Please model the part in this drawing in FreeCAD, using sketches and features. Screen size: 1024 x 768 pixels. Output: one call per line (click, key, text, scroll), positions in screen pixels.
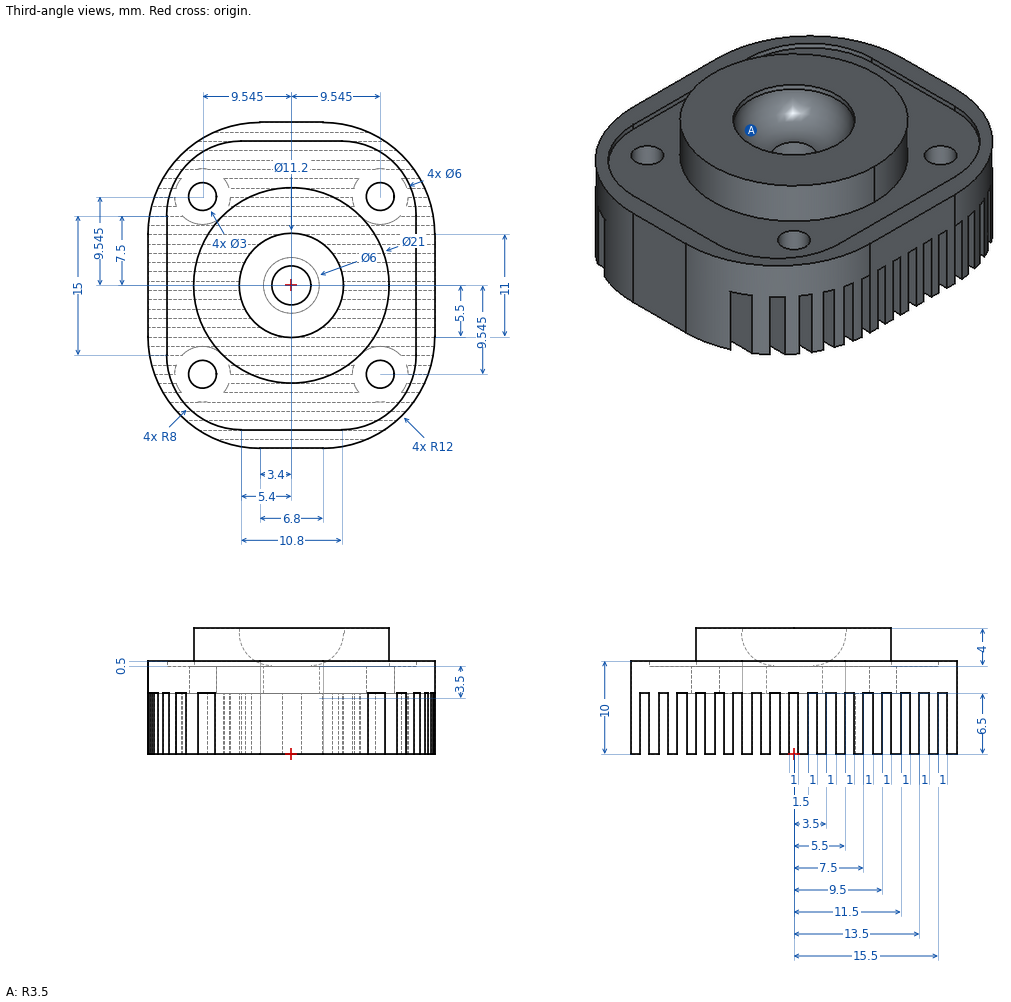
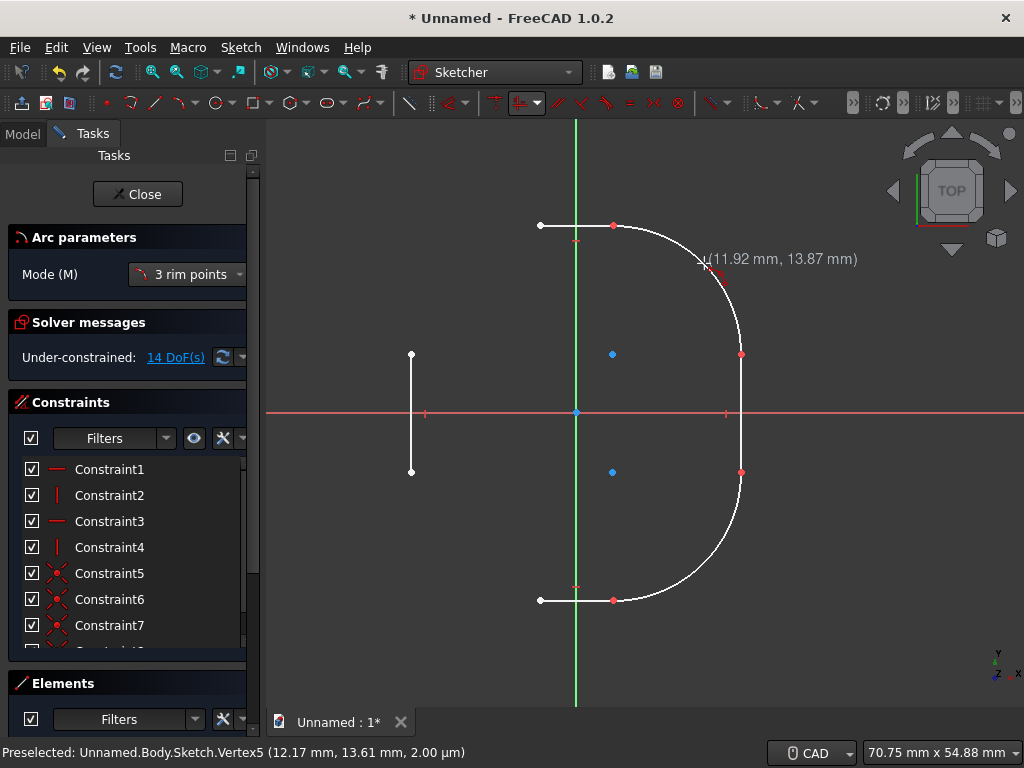
click(540, 226)
click(411, 355)
click(449, 263)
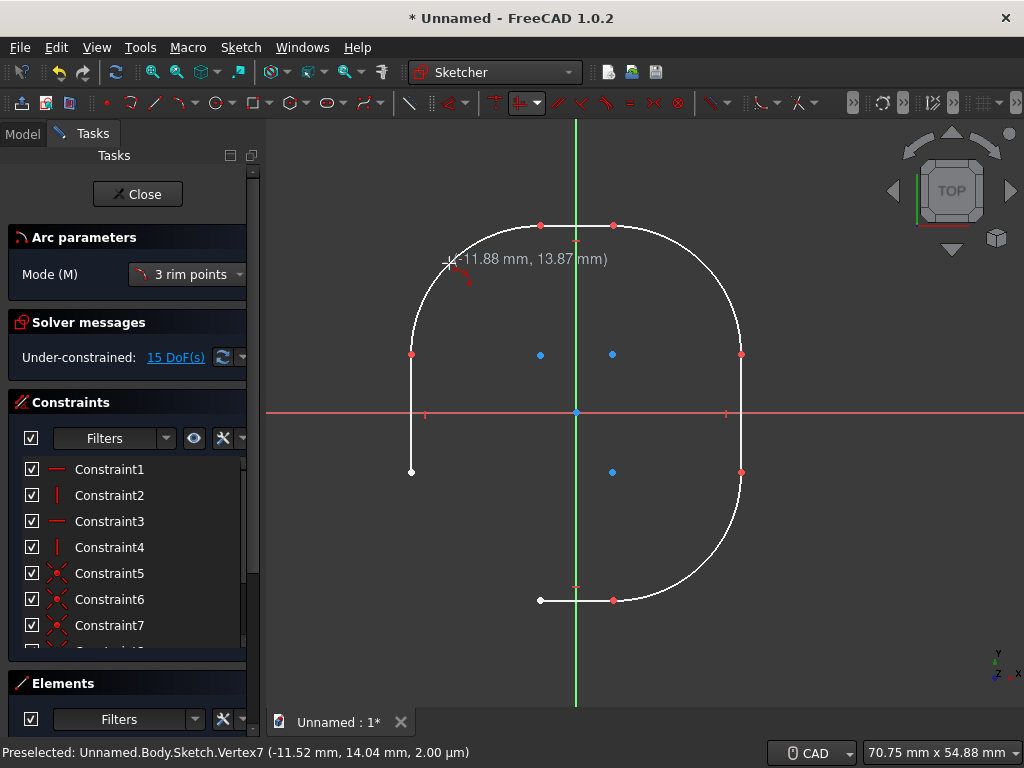
click(411, 473)
click(540, 601)
click(449, 562)
key(Escape)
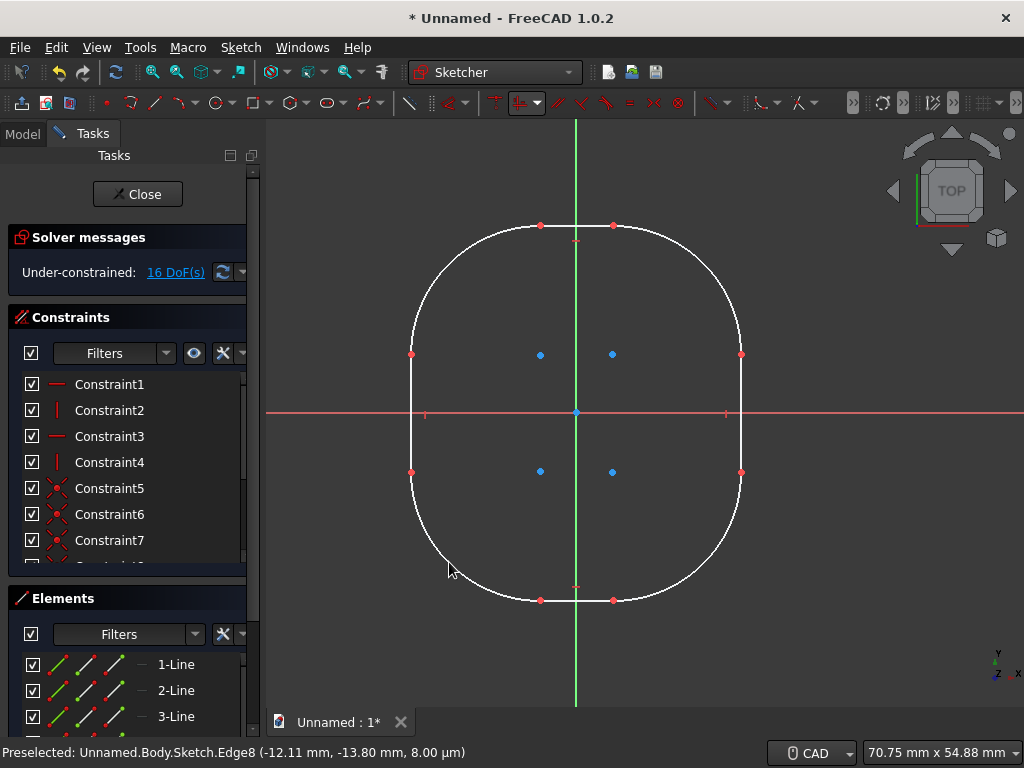
click(562, 601)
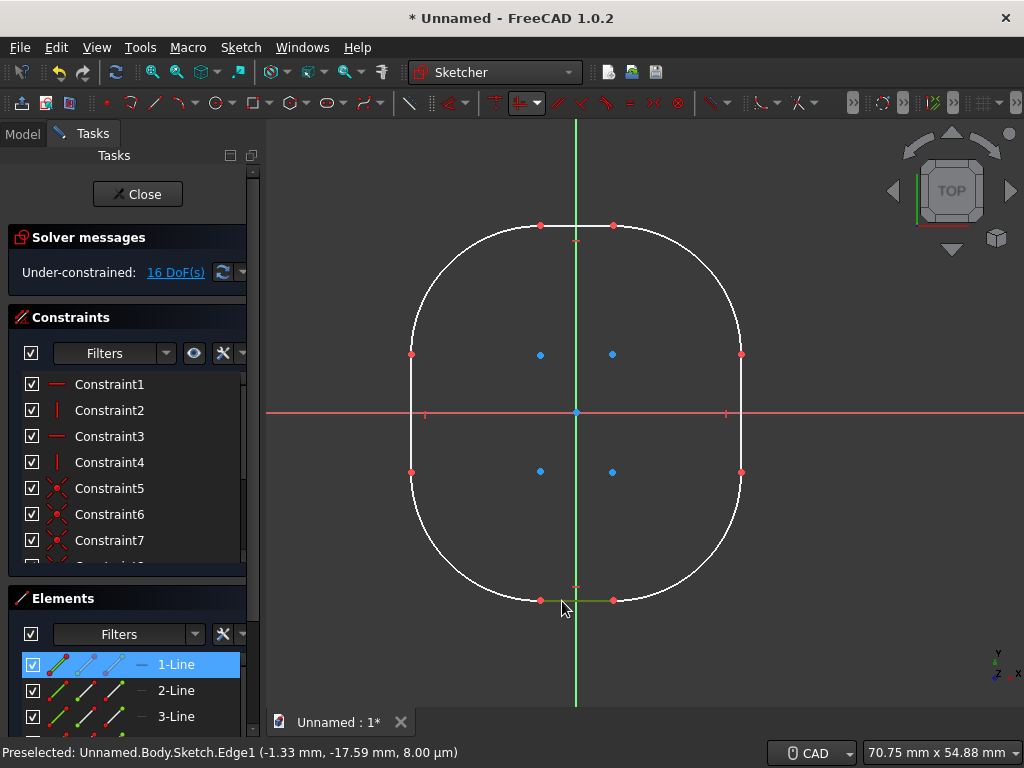
click(671, 587)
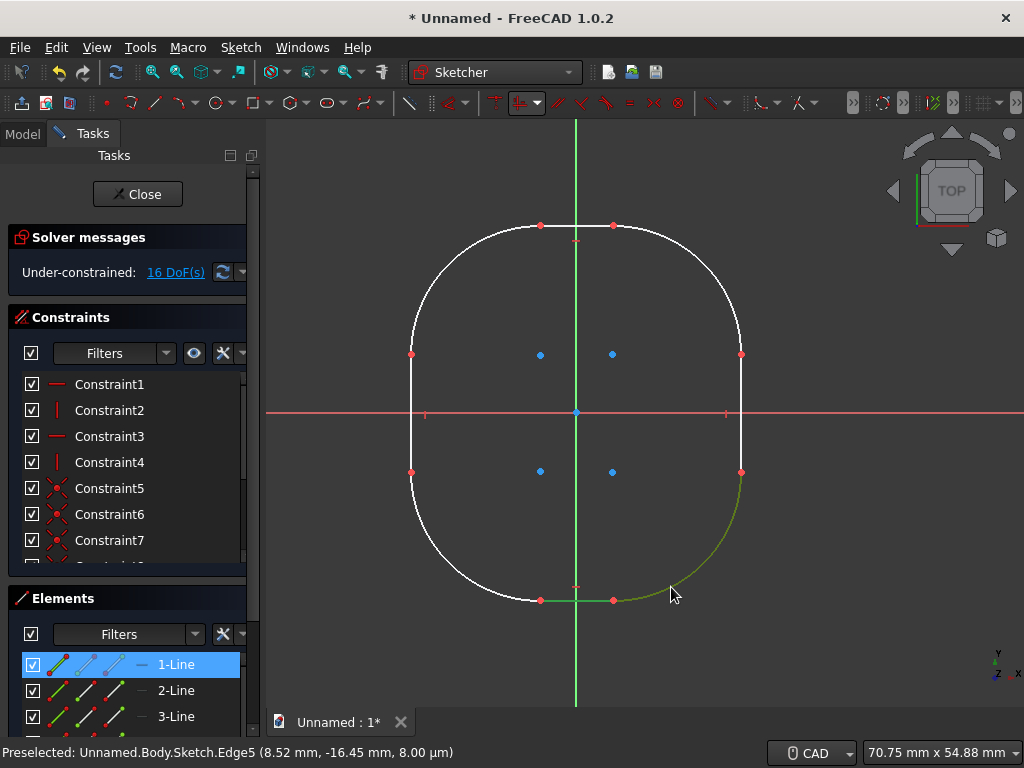
key(t)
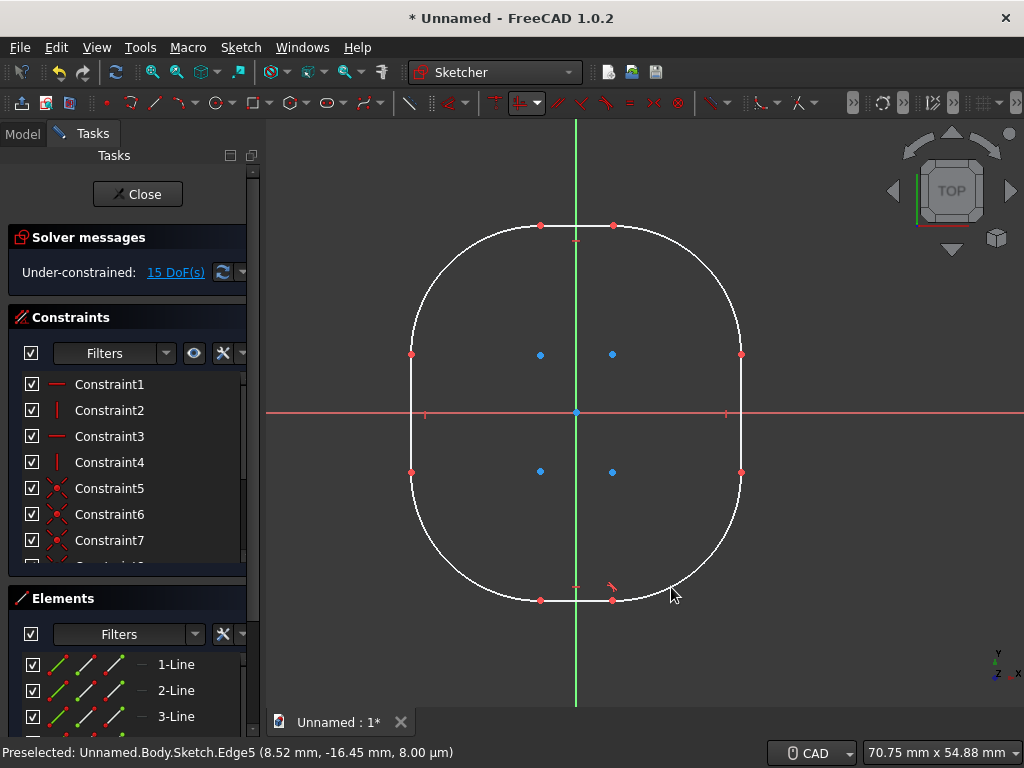
click(562, 601)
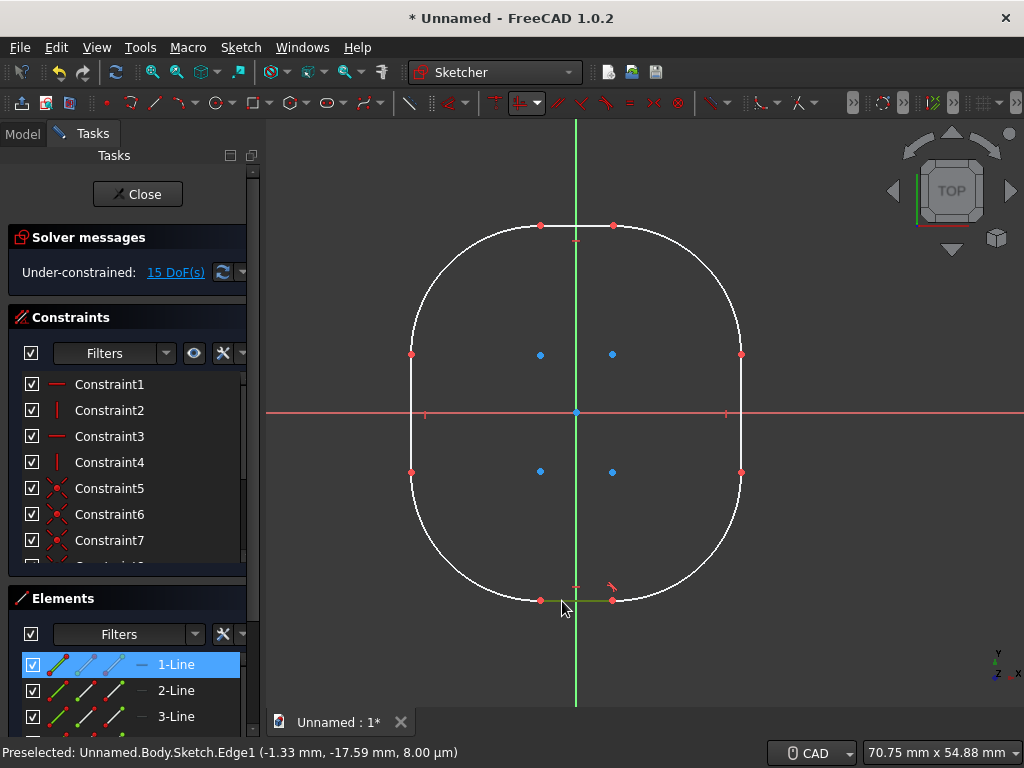
click(426, 531)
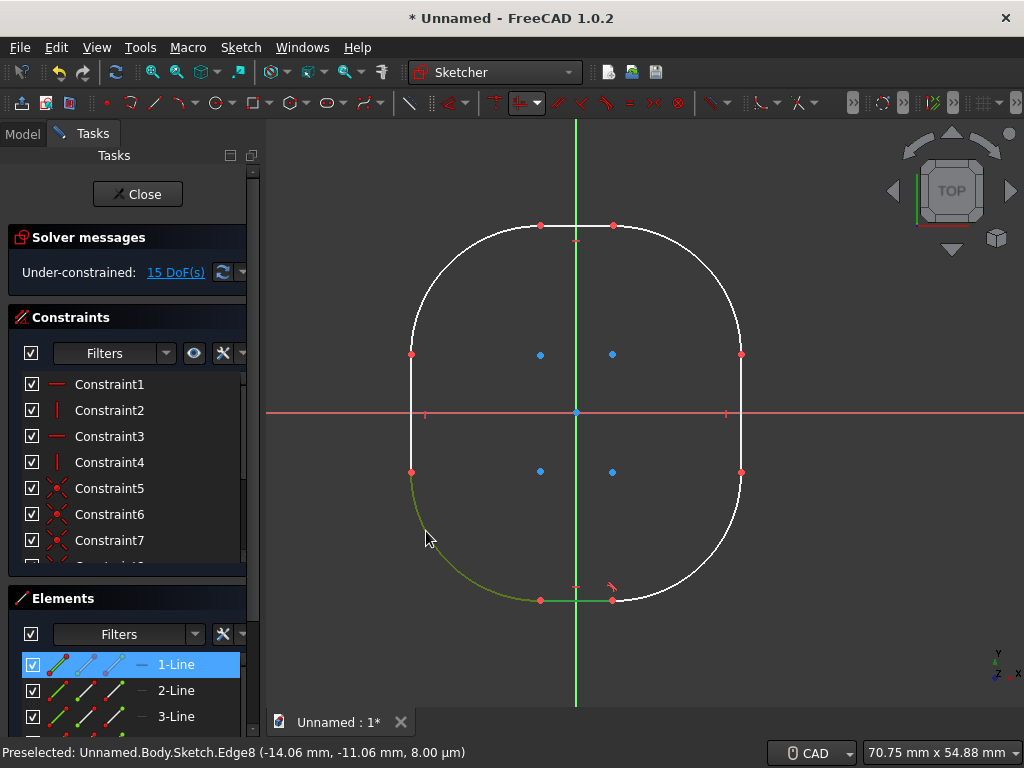
click(606, 104)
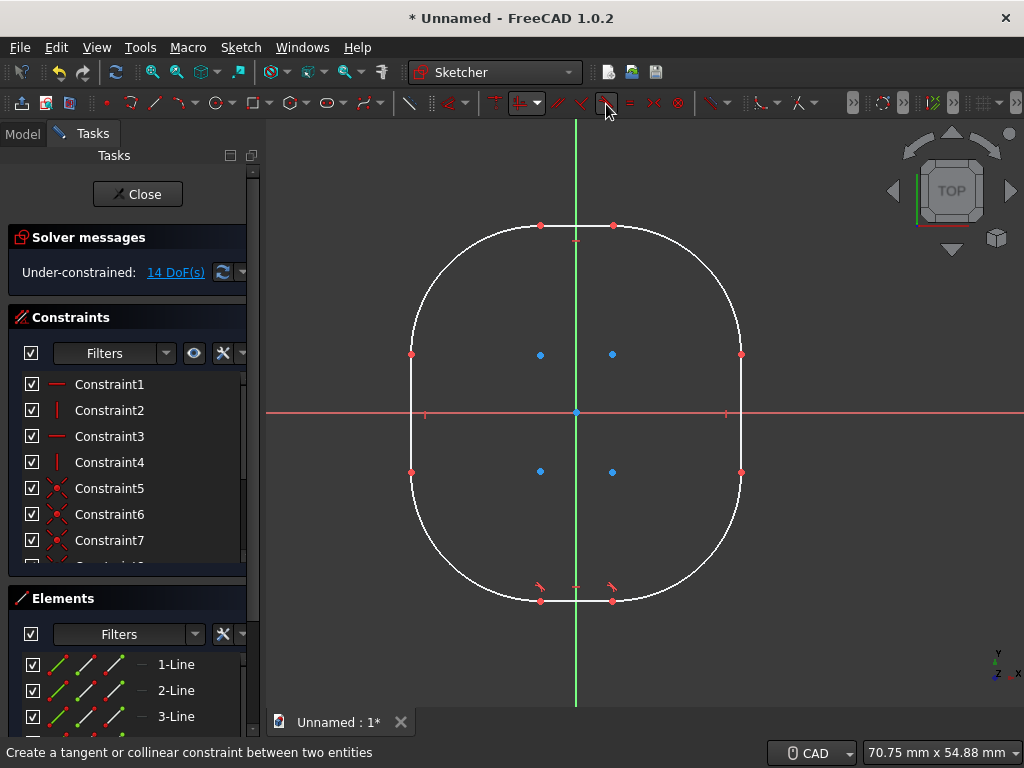
click(741, 438)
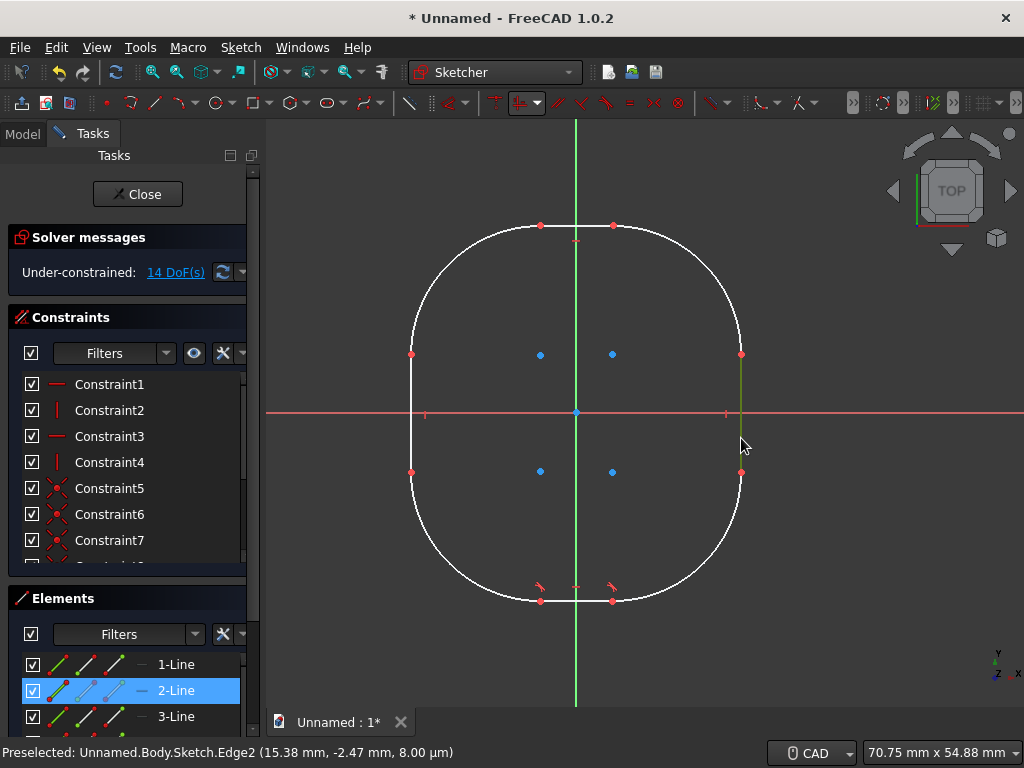
click(671, 587)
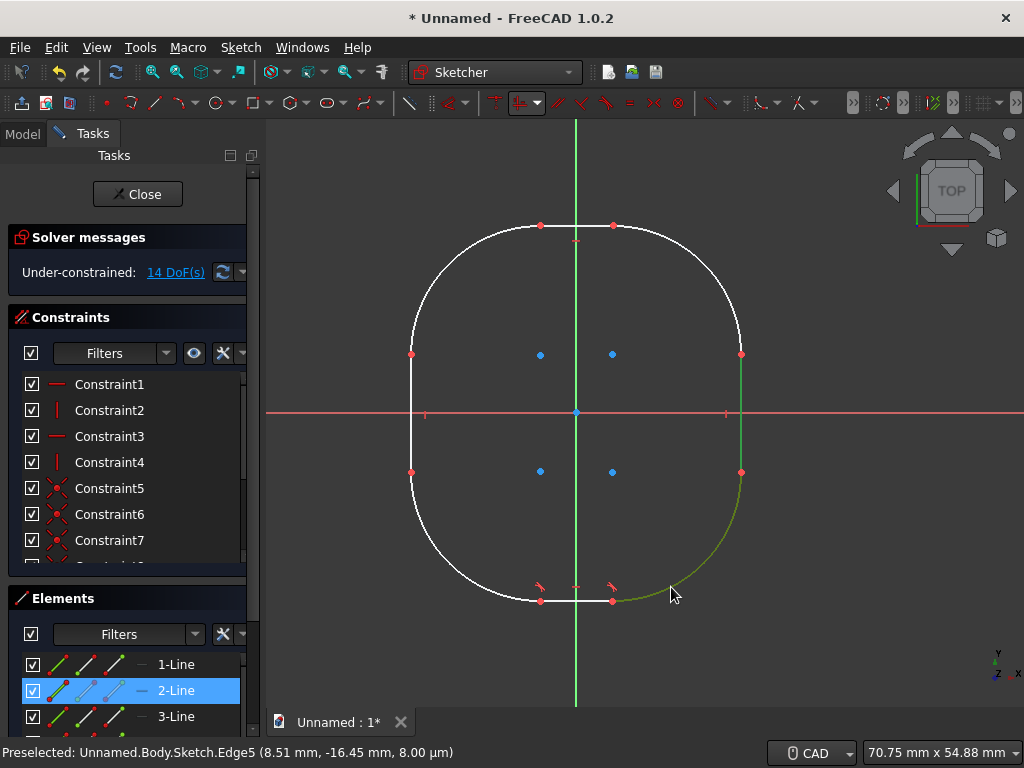
click(606, 104)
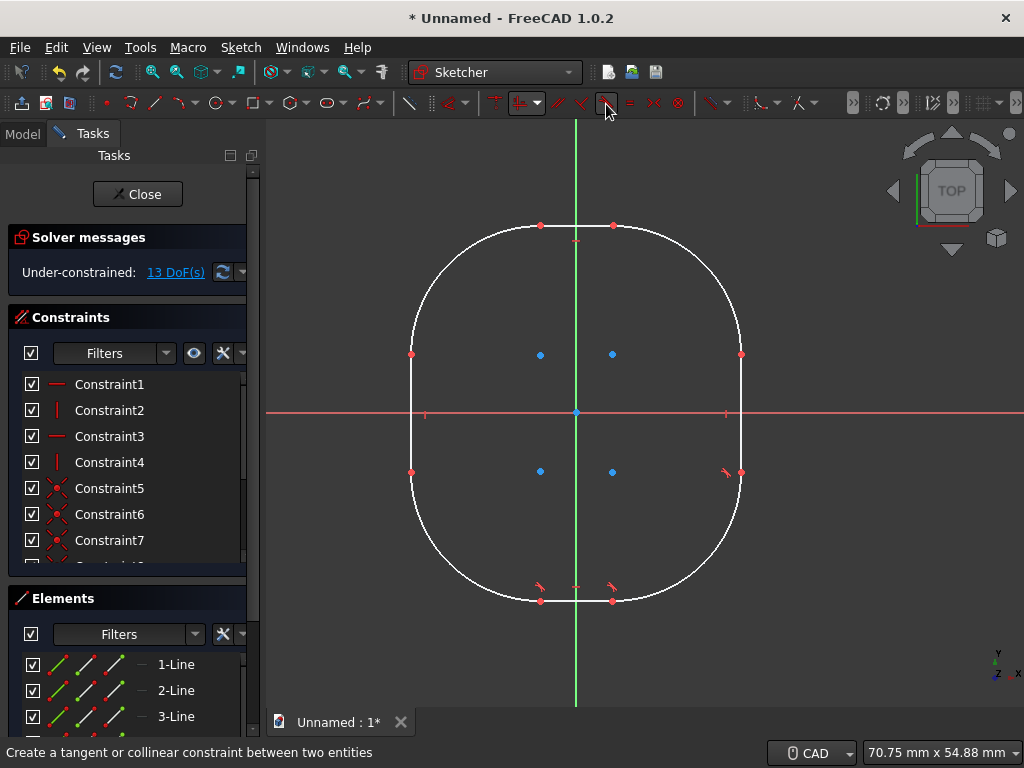
click(741, 438)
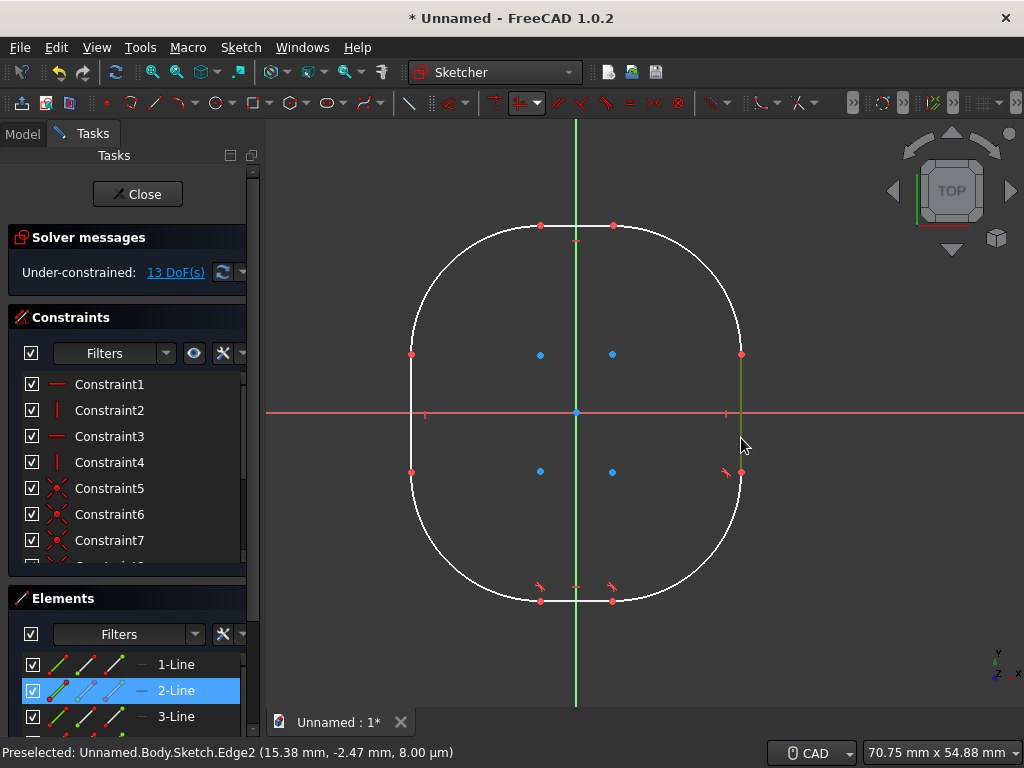
click(727, 297)